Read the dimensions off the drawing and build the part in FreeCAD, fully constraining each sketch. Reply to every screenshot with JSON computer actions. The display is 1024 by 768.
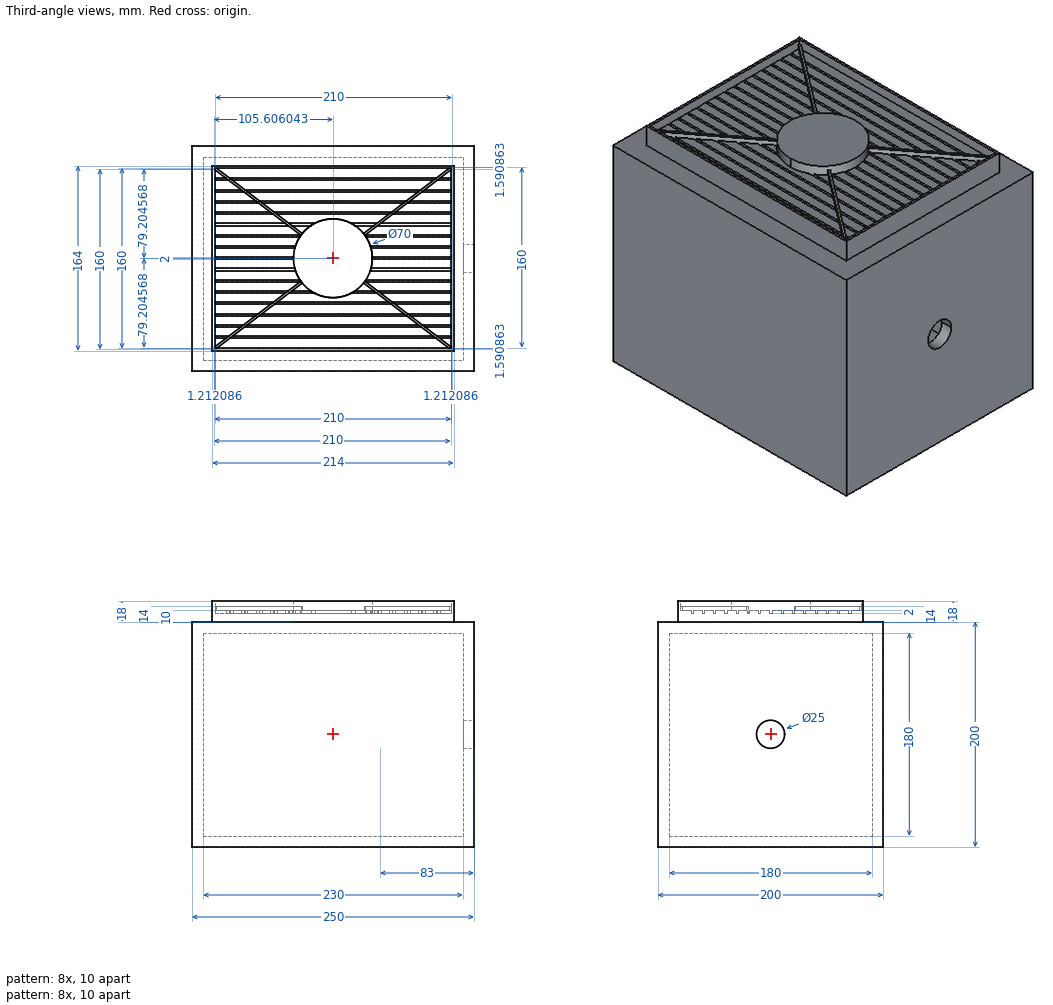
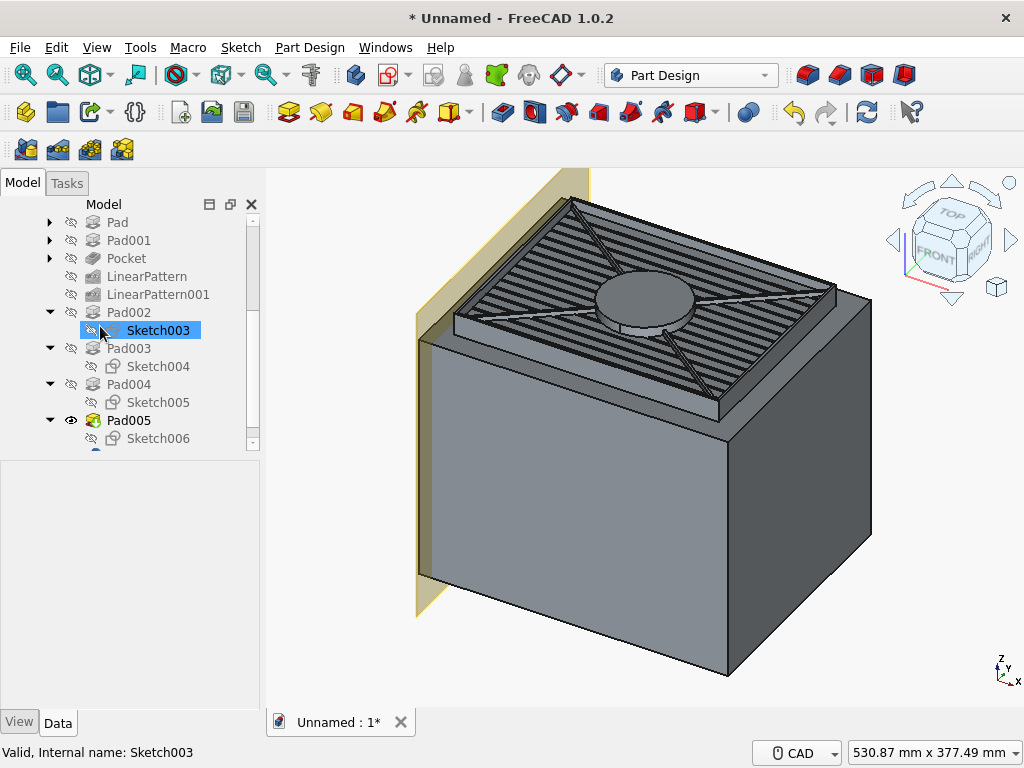
{"action": "scroll", "coordinate": [140, 326], "scroll_direction": "up", "scroll_amount": 15}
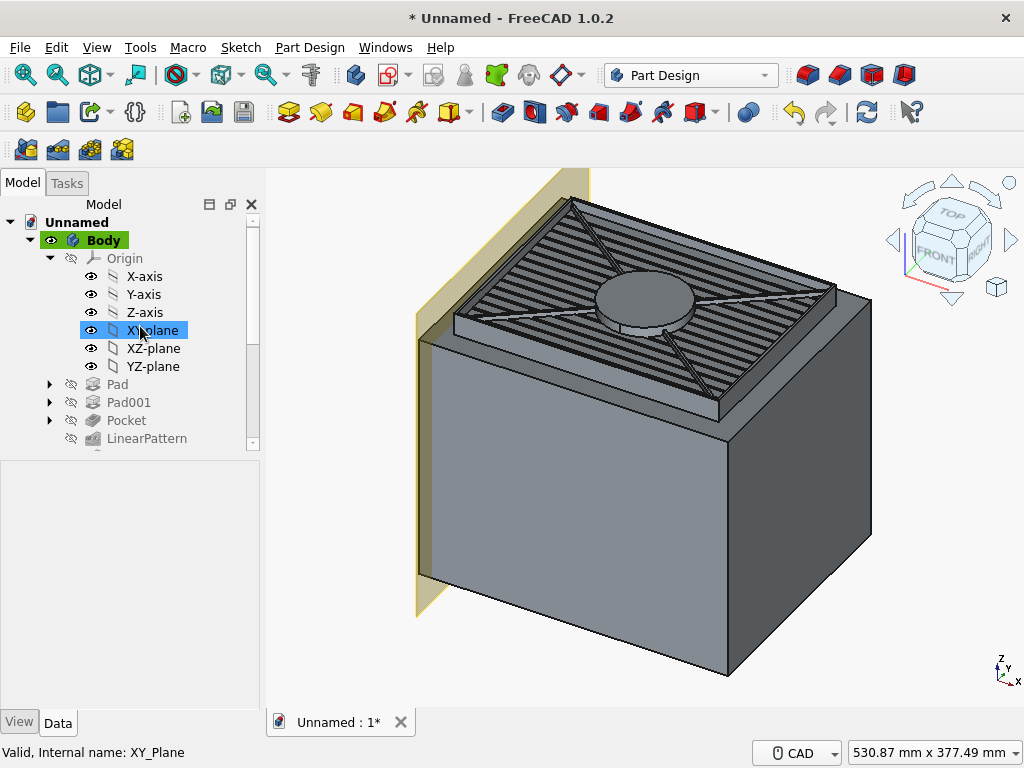
{"action": "scroll", "coordinate": [100, 326], "scroll_direction": "down", "scroll_amount": 6}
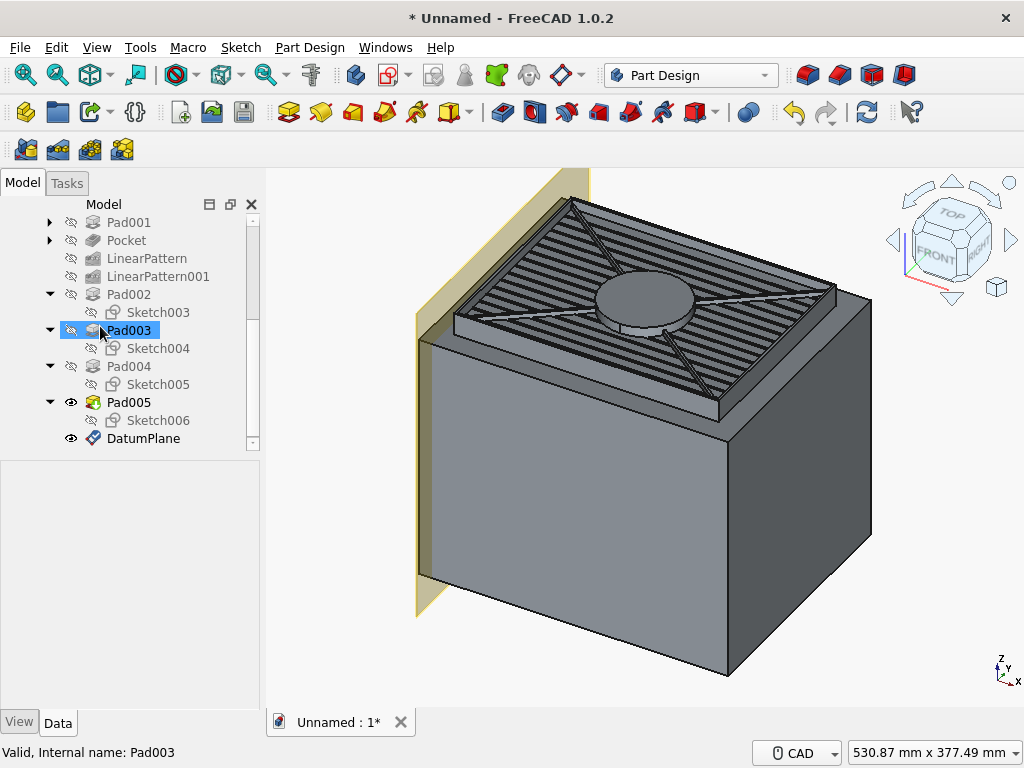
{"action": "left_click", "coordinate": [116, 438]}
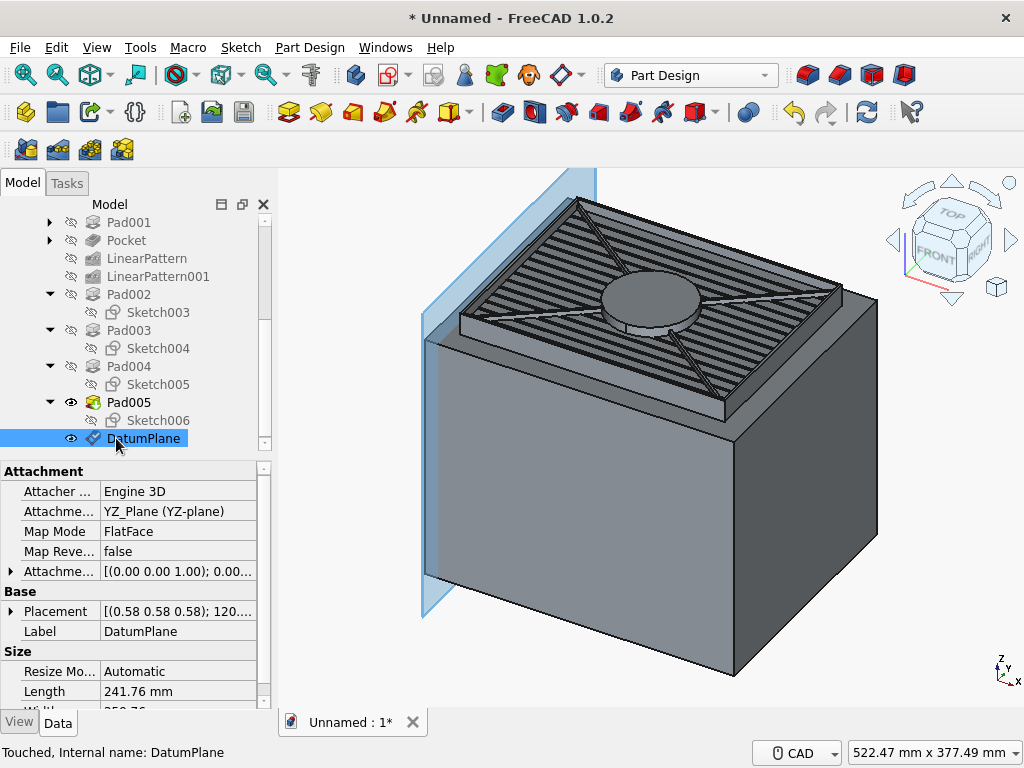
{"action": "left_click", "coordinate": [388, 76]}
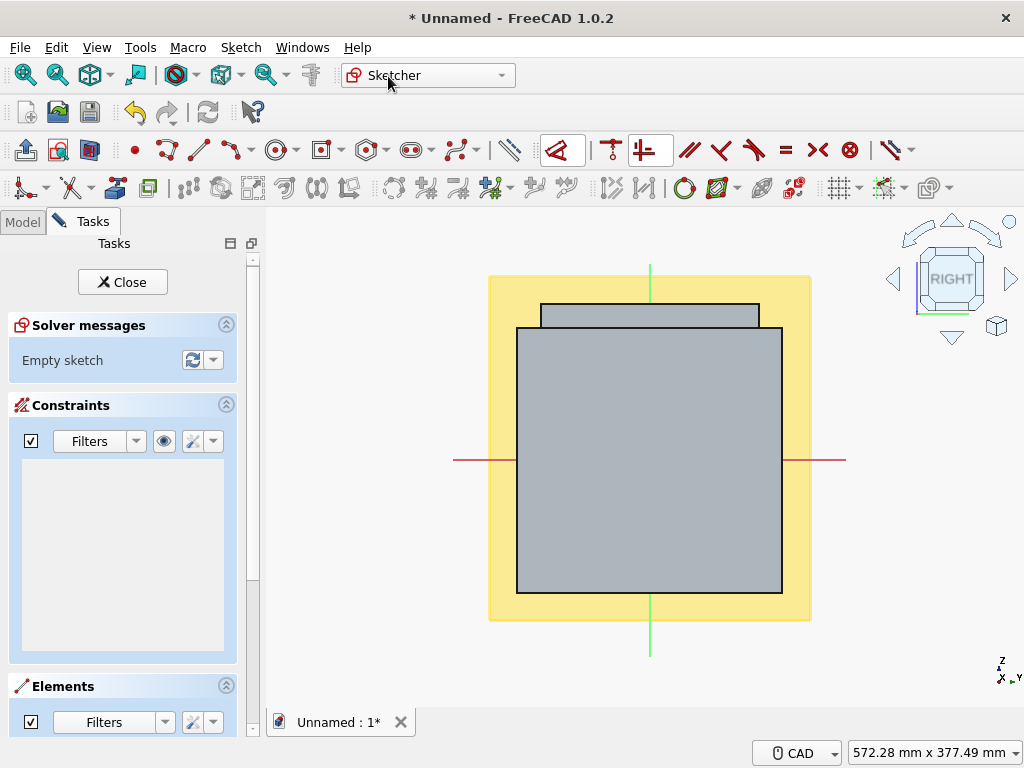
{"action": "left_click", "coordinate": [90, 150]}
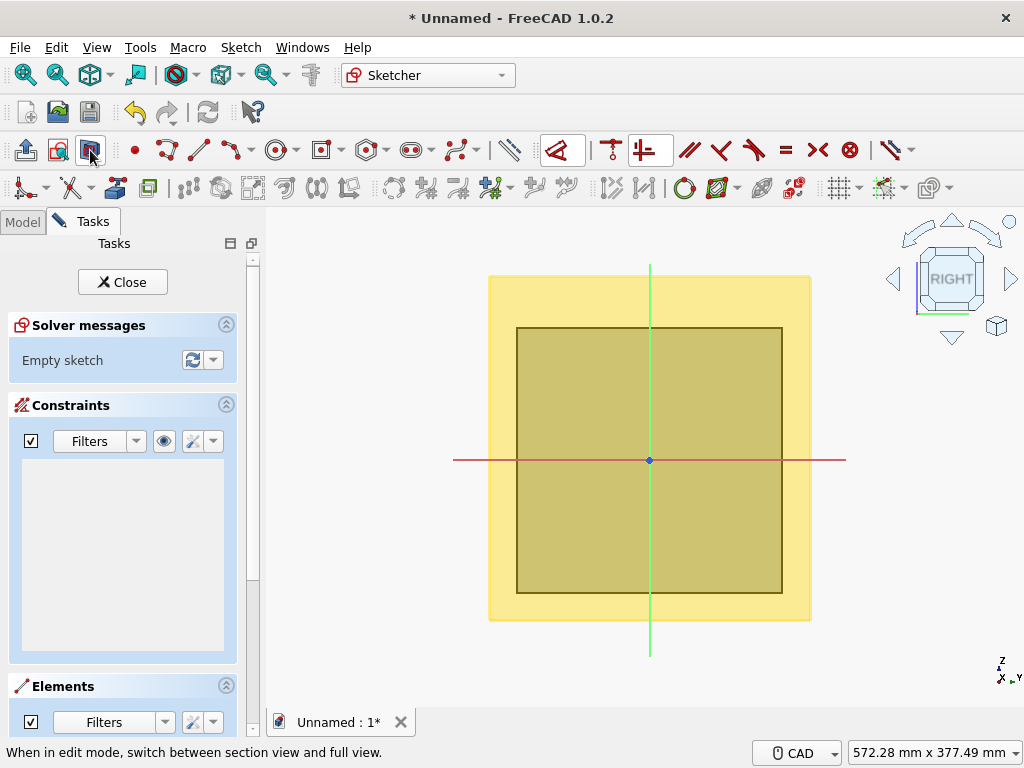
{"action": "left_click", "coordinate": [322, 150]}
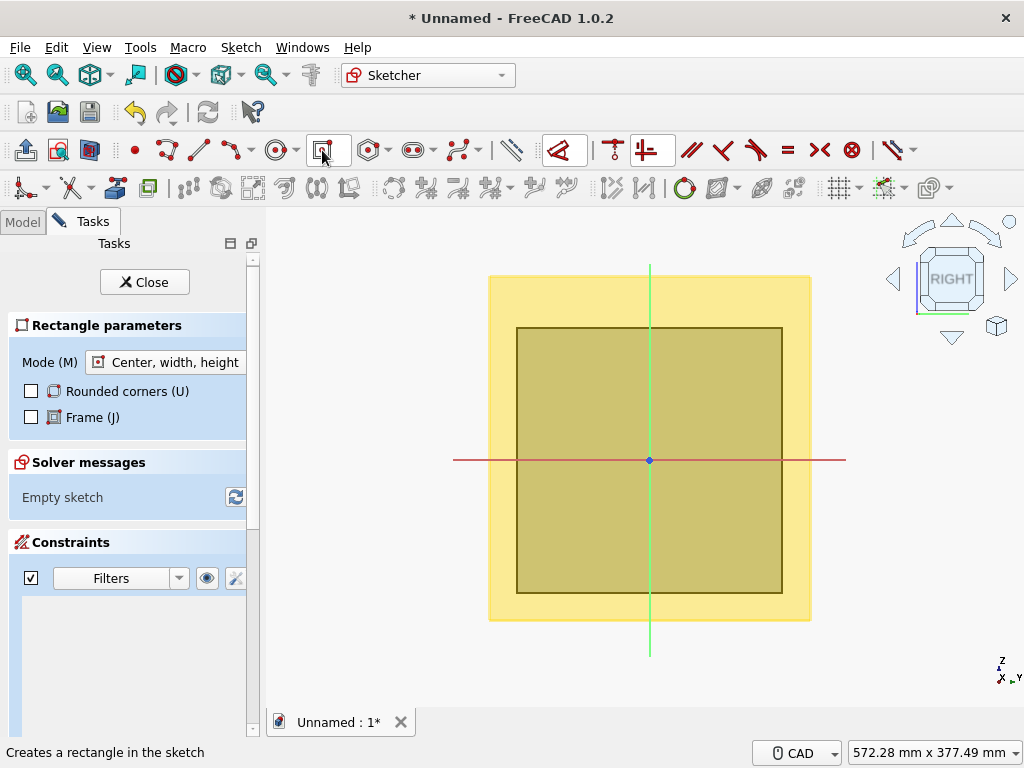
{"action": "left_click", "coordinate": [650, 460]}
{"action": "left_click", "coordinate": [769, 341]}
{"action": "key", "text": "Escape"}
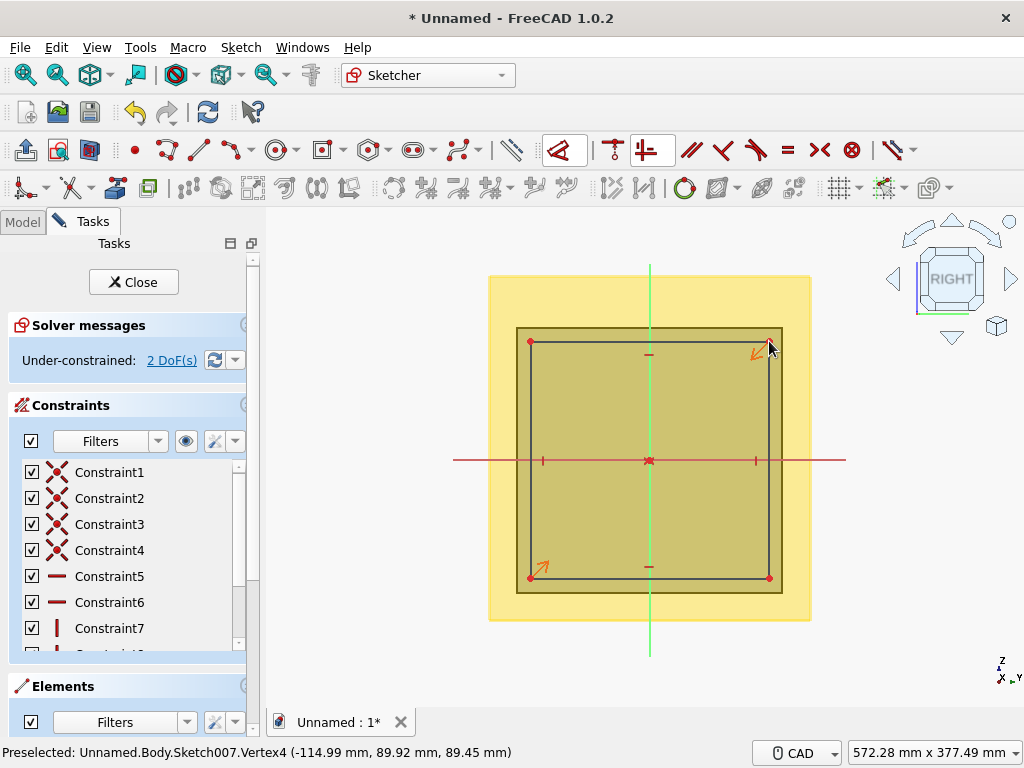
{"action": "left_click", "coordinate": [602, 579]}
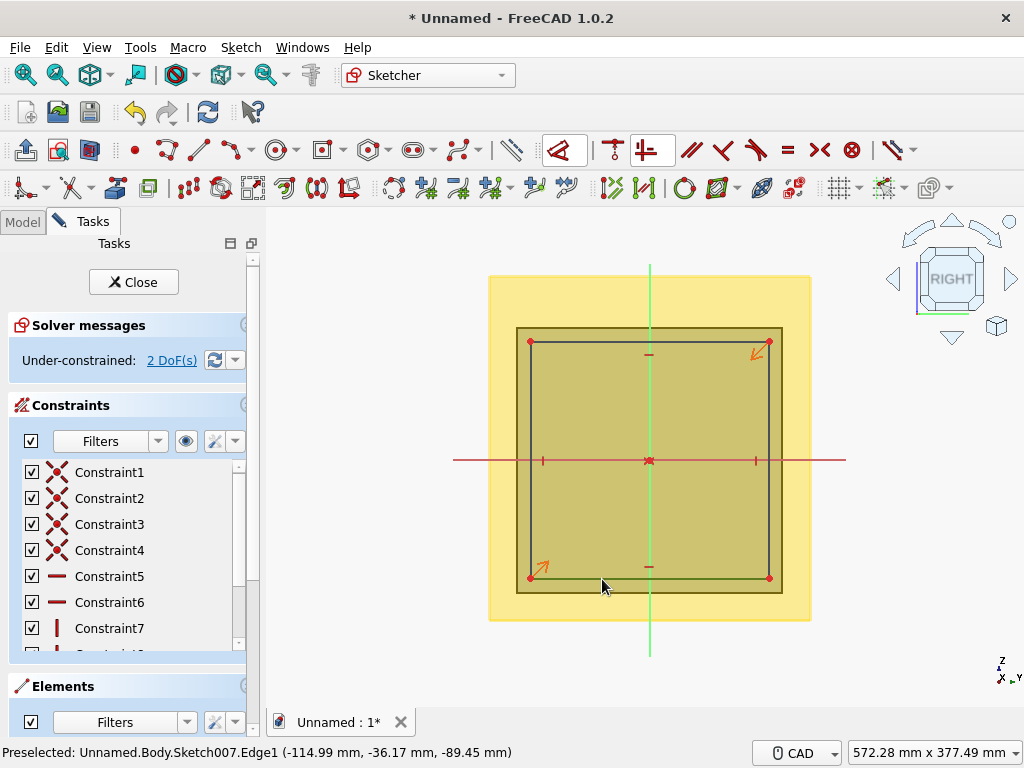
{"action": "left_click", "coordinate": [582, 150]}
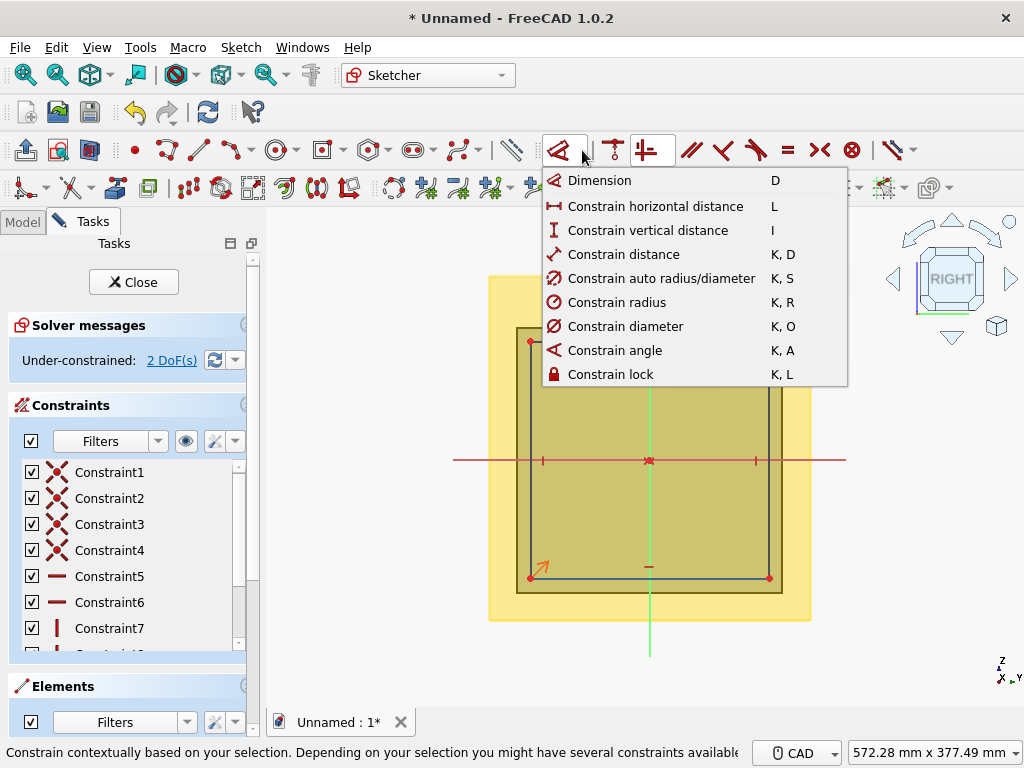
{"action": "left_click", "coordinate": [695, 206]}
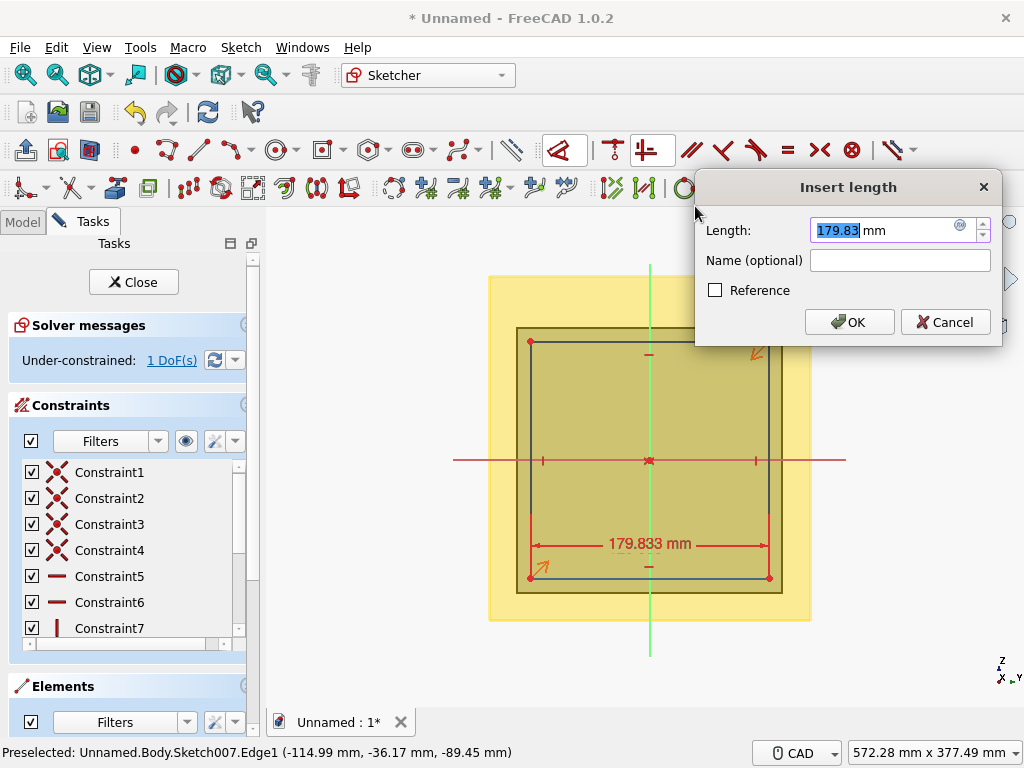
{"action": "type", "text": "180"}
{"action": "key", "text": "Return"}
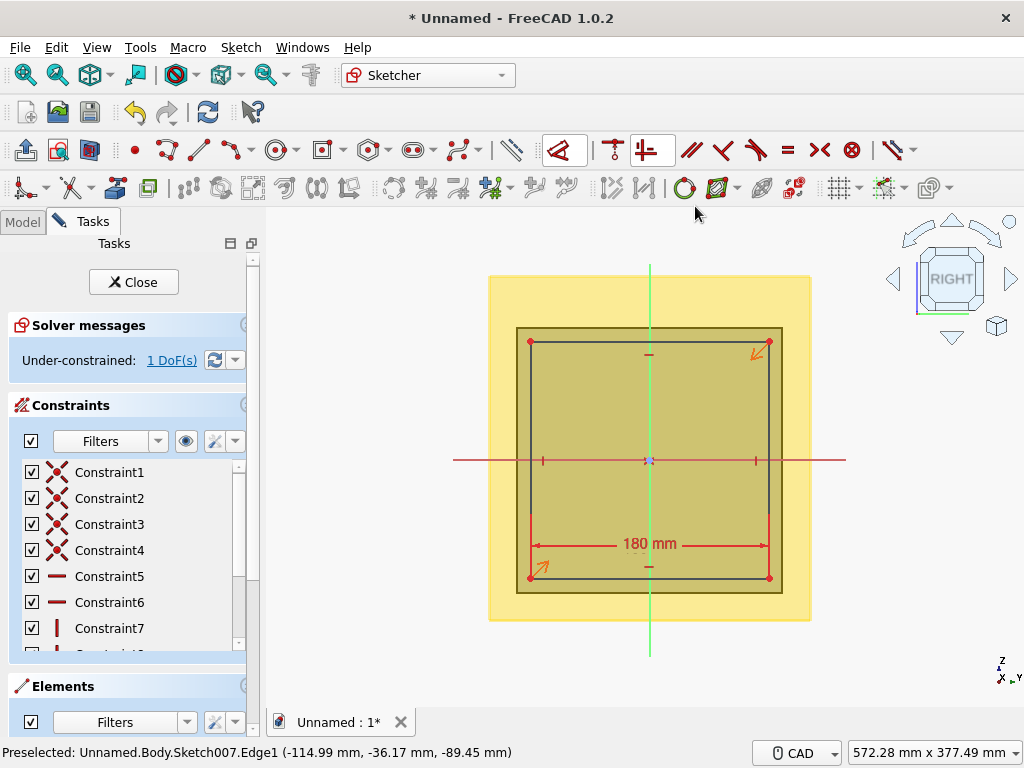
{"action": "left_click", "coordinate": [769, 508]}